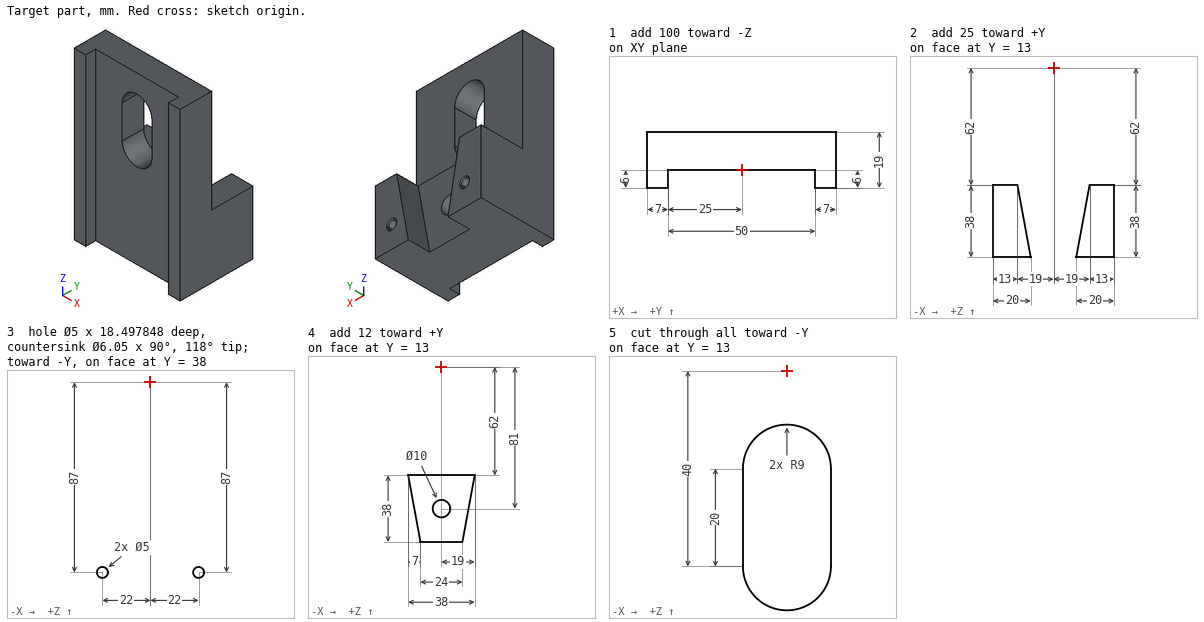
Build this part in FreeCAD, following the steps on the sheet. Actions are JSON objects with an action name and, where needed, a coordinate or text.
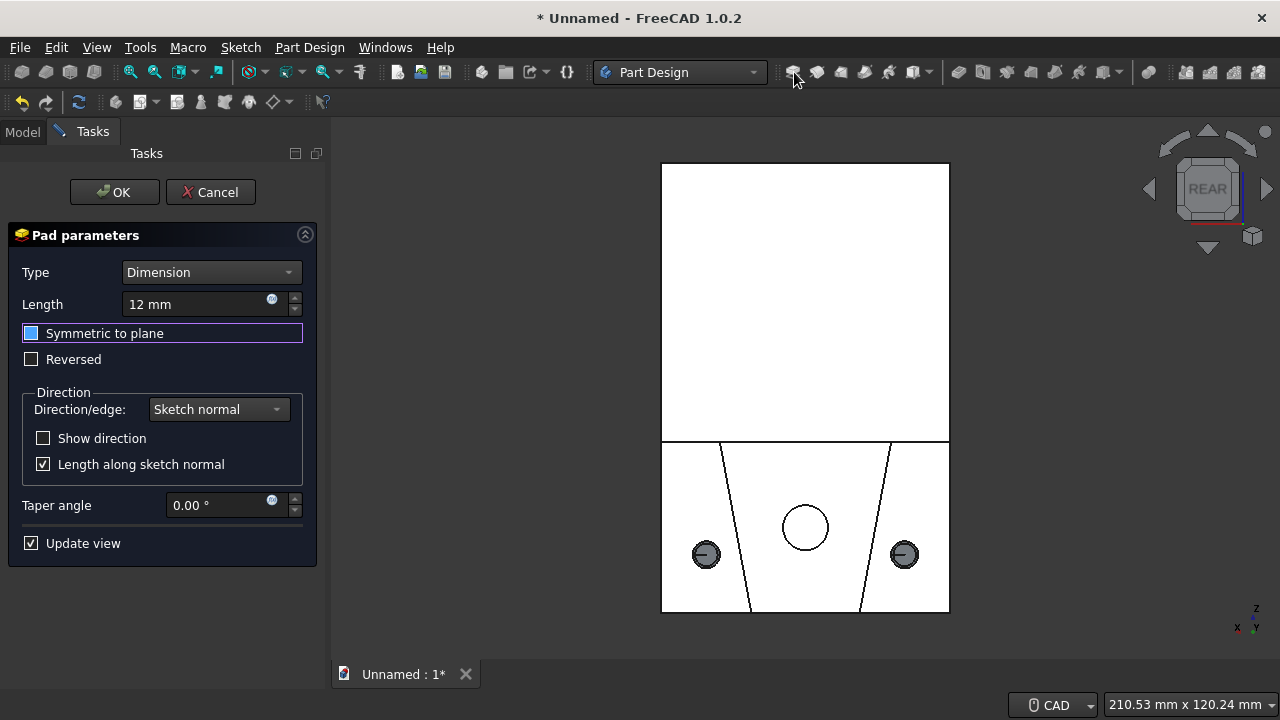
{"action": "left_click", "coordinate": [115, 192]}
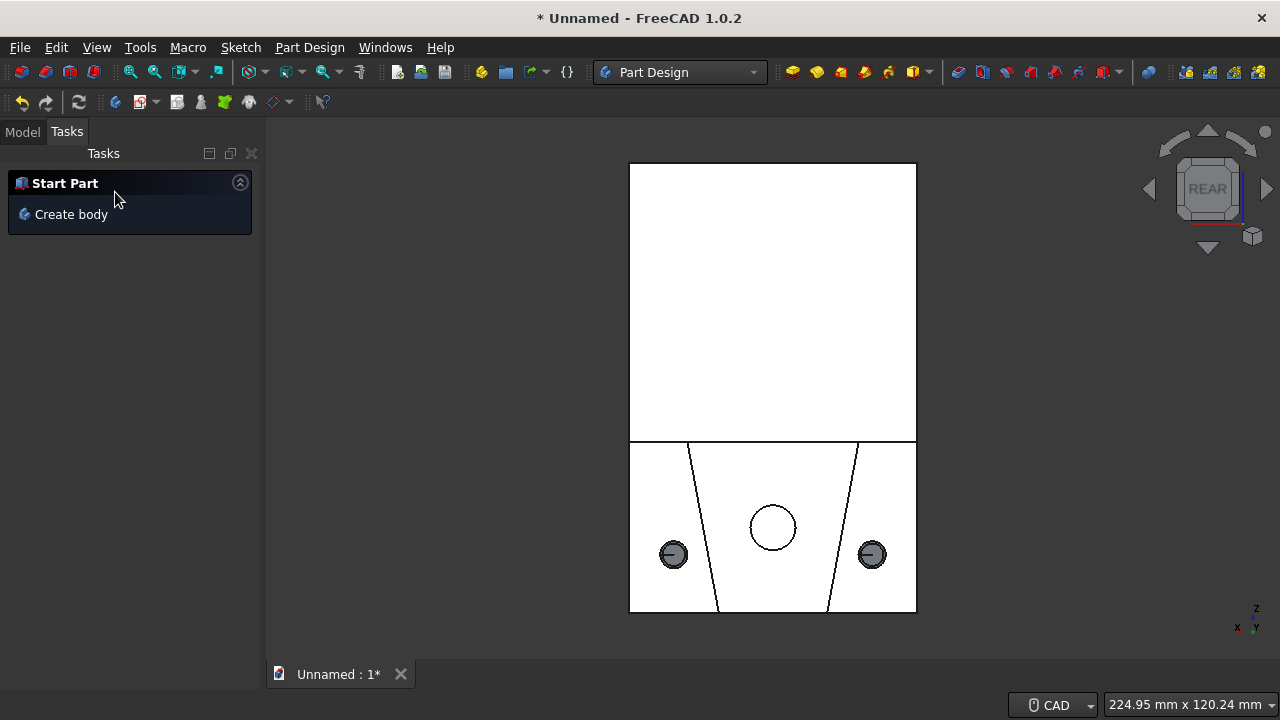
{"action": "left_click", "coordinate": [773, 301]}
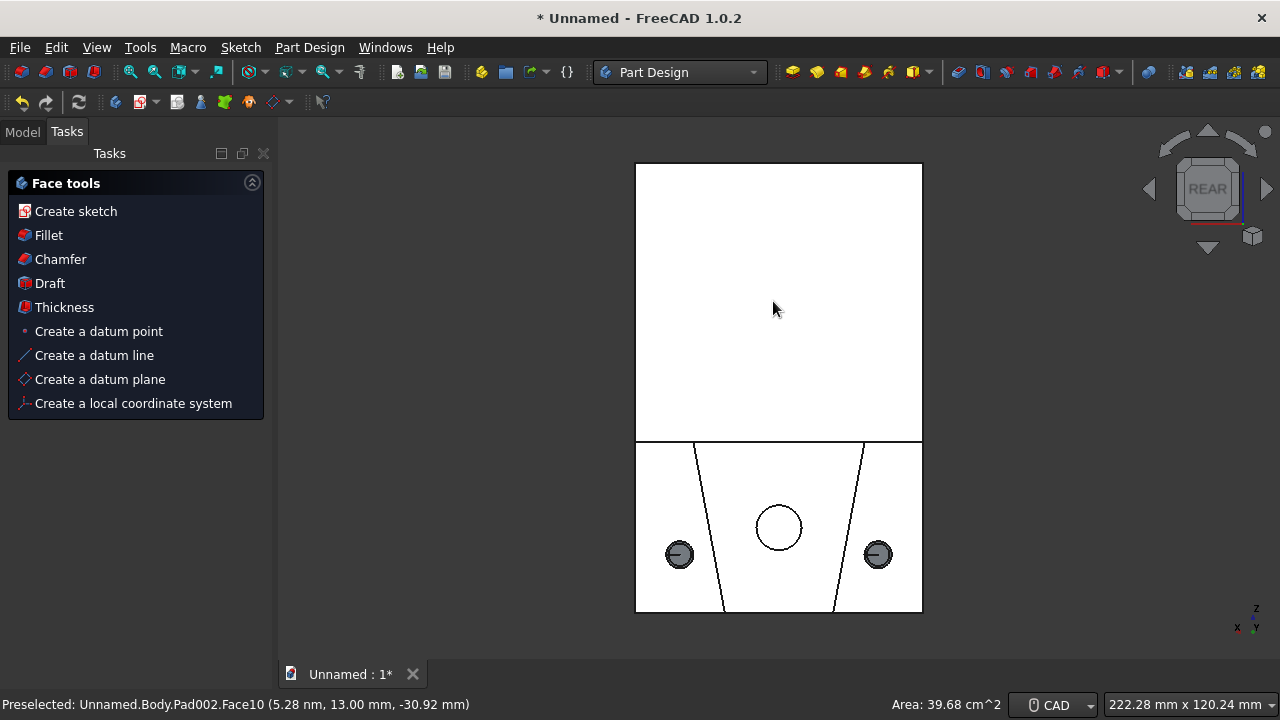
{"action": "left_click", "coordinate": [140, 102]}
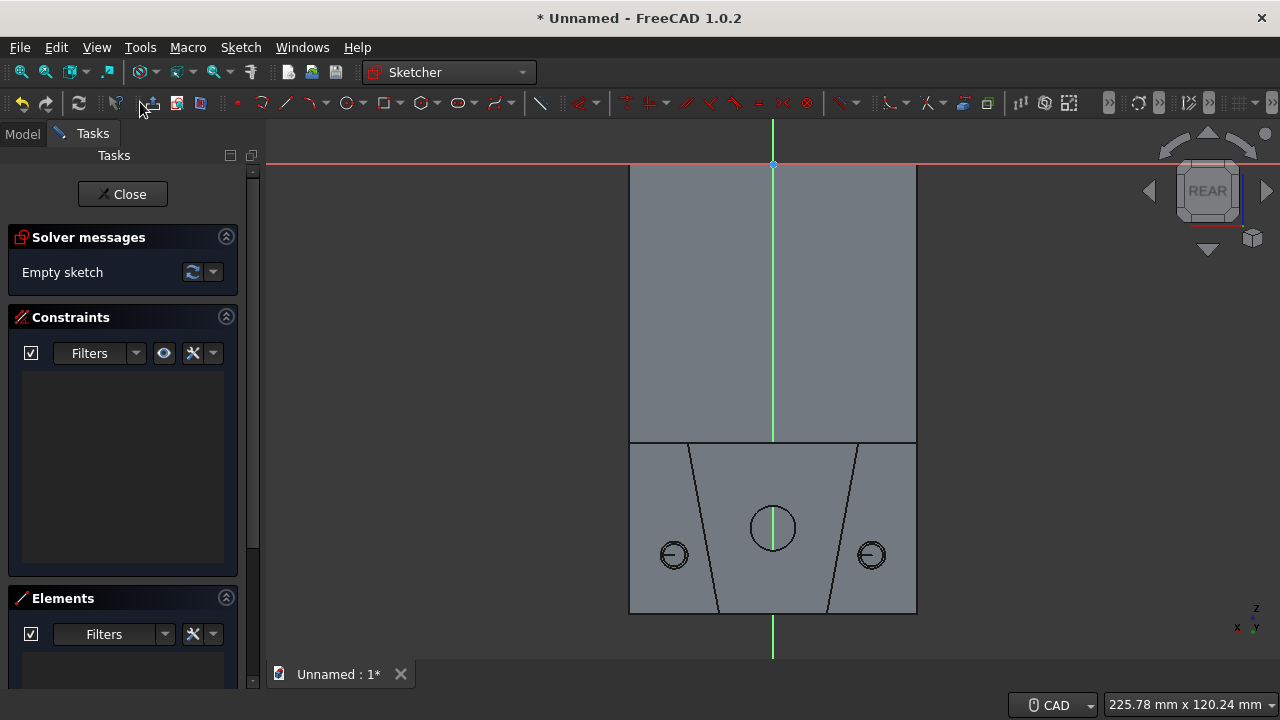
{"action": "key", "text": "q s"}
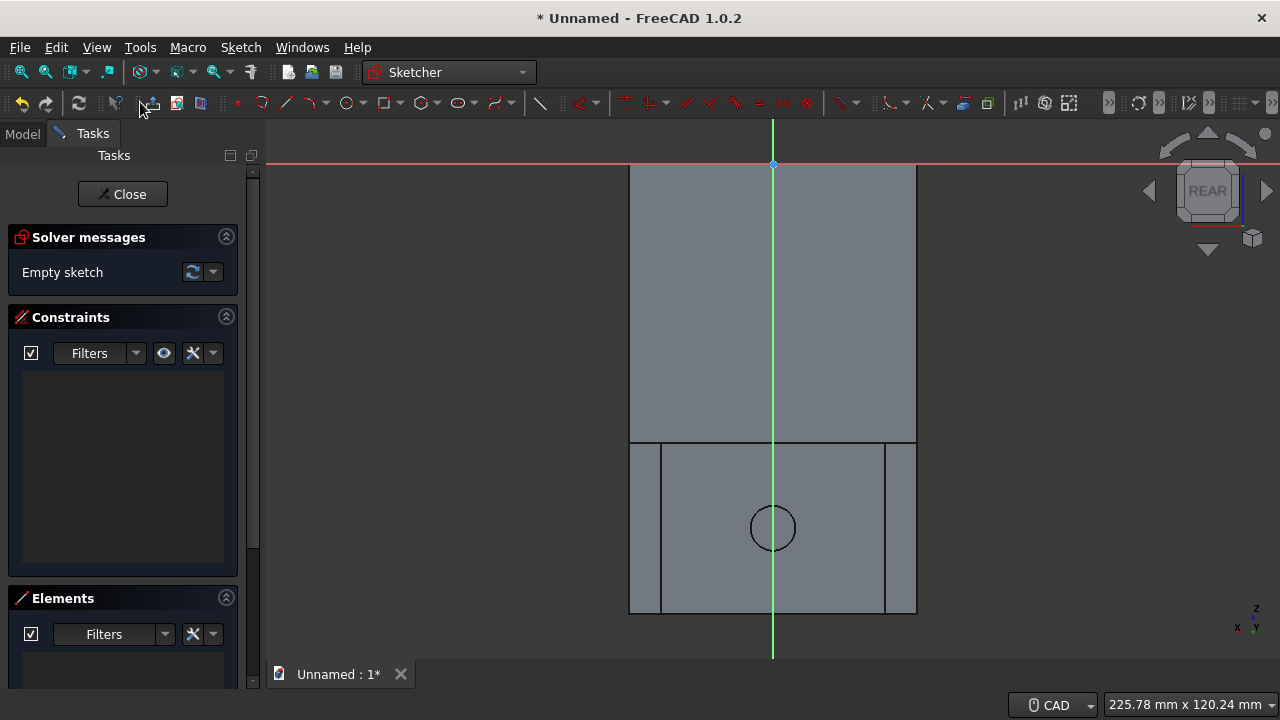
{"action": "scroll", "coordinate": [912, 147], "scroll_direction": "up", "scroll_amount": 2}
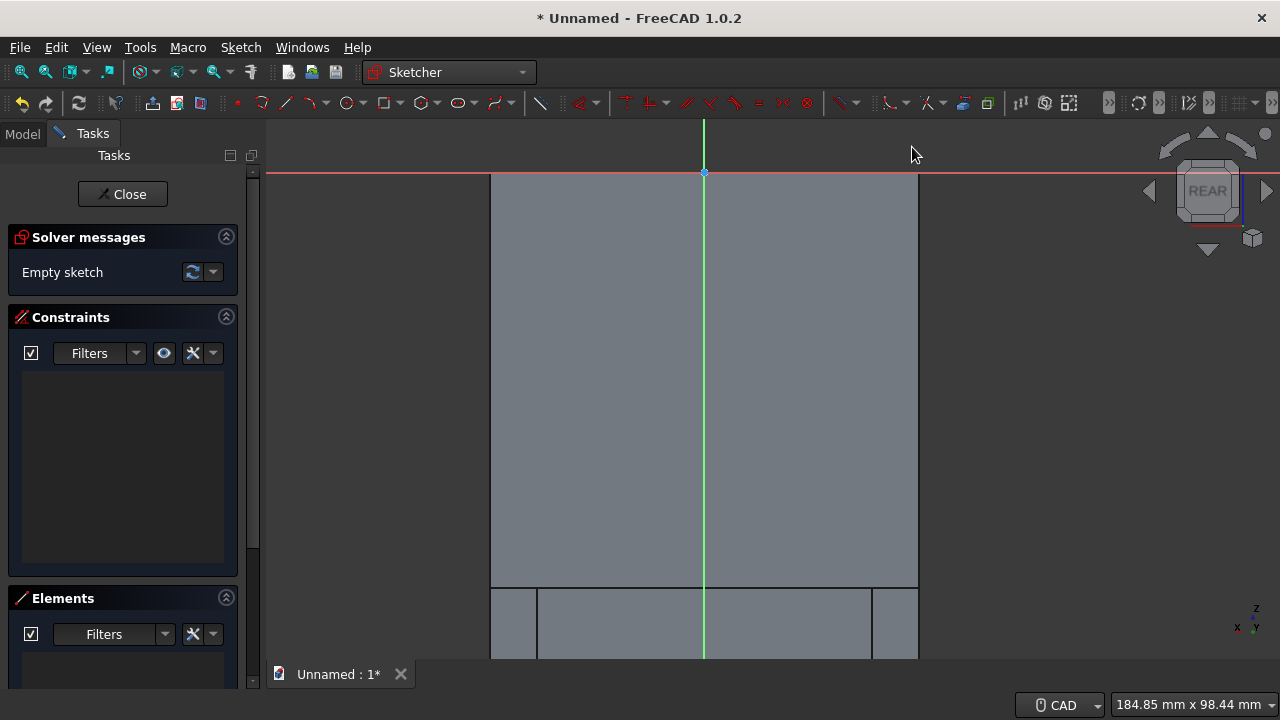
{"action": "left_click", "coordinate": [458, 104]}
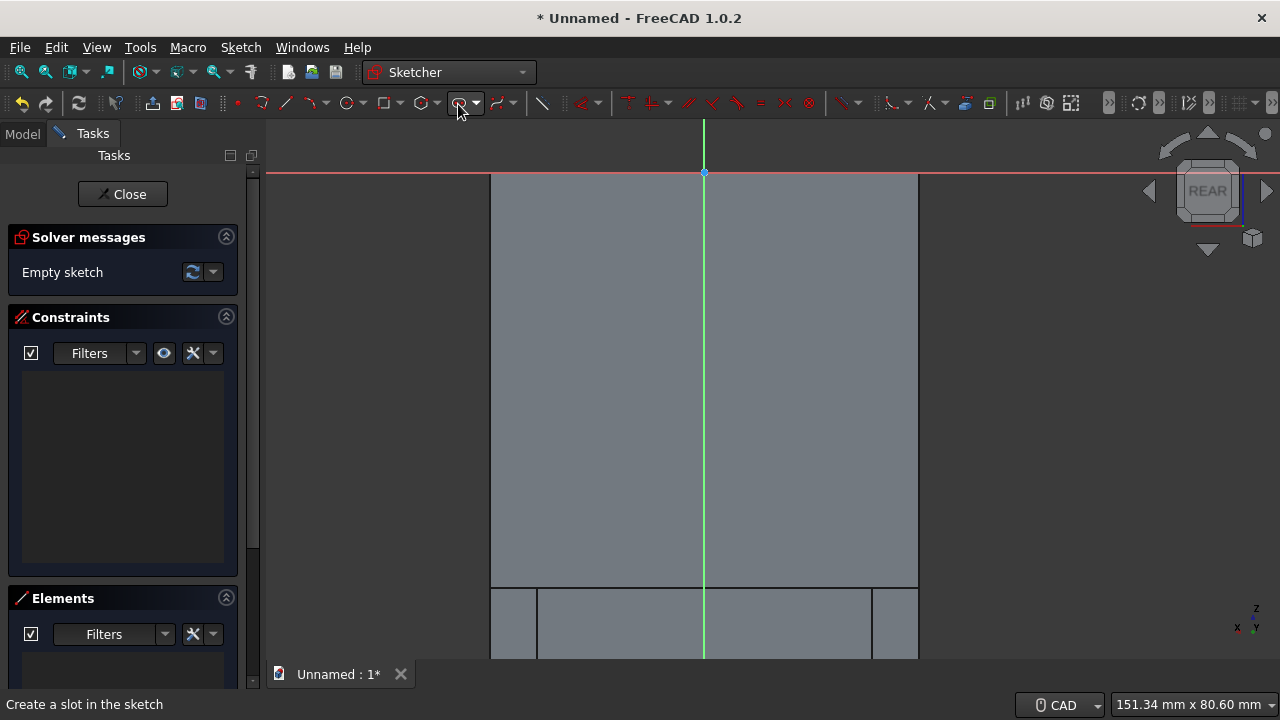
{"action": "left_click", "coordinate": [704, 441]}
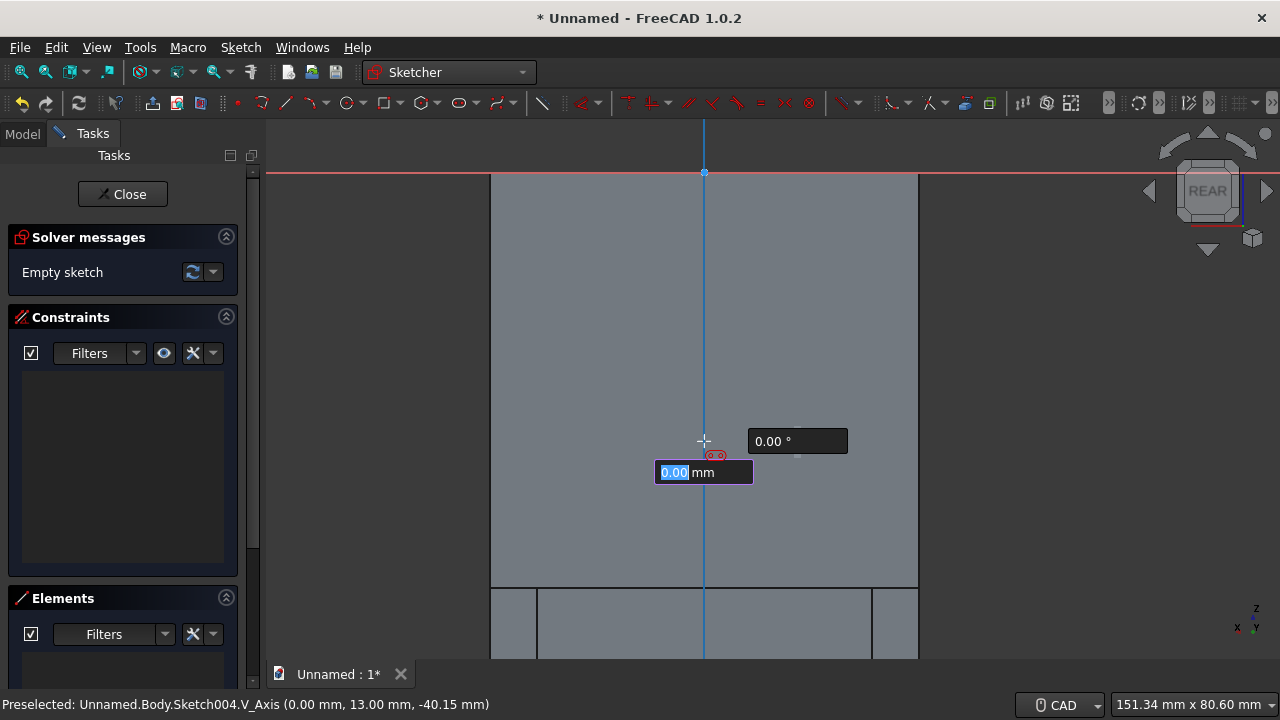
{"action": "left_click", "coordinate": [713, 307]}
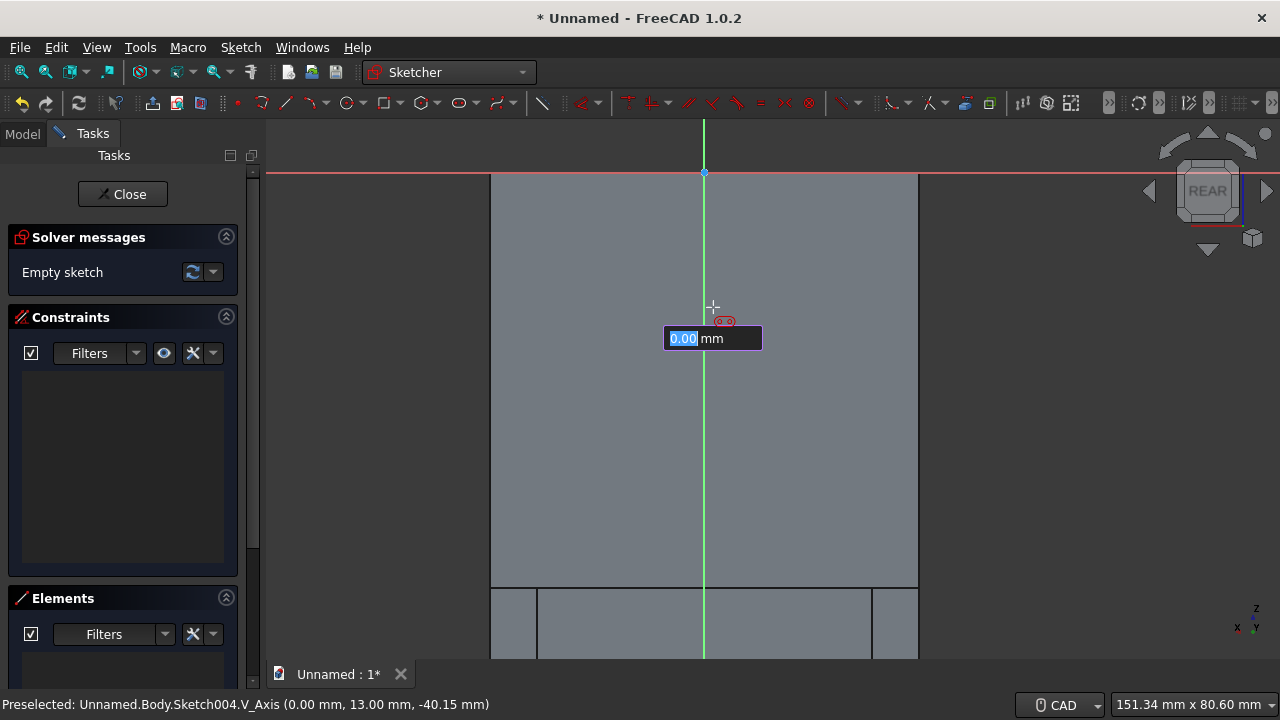
{"action": "left_click", "coordinate": [765, 374]}
{"action": "key", "text": "Escape"}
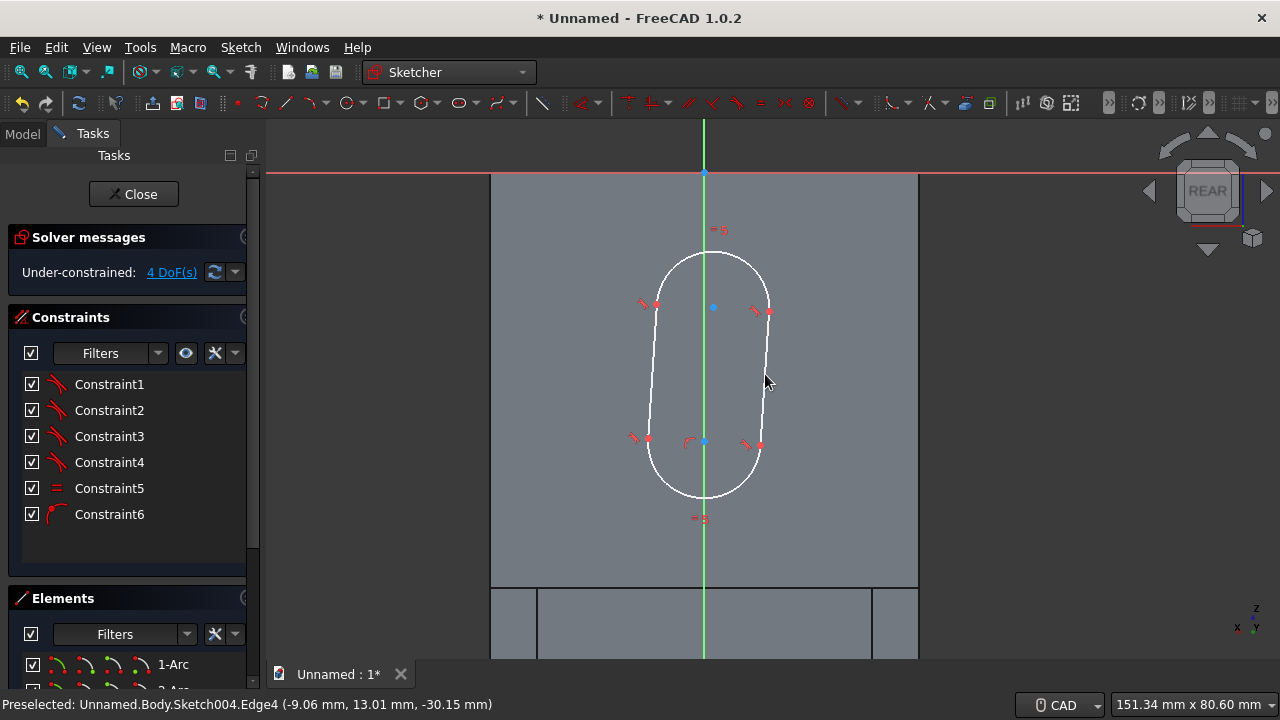
{"action": "left_click", "coordinate": [651, 398]}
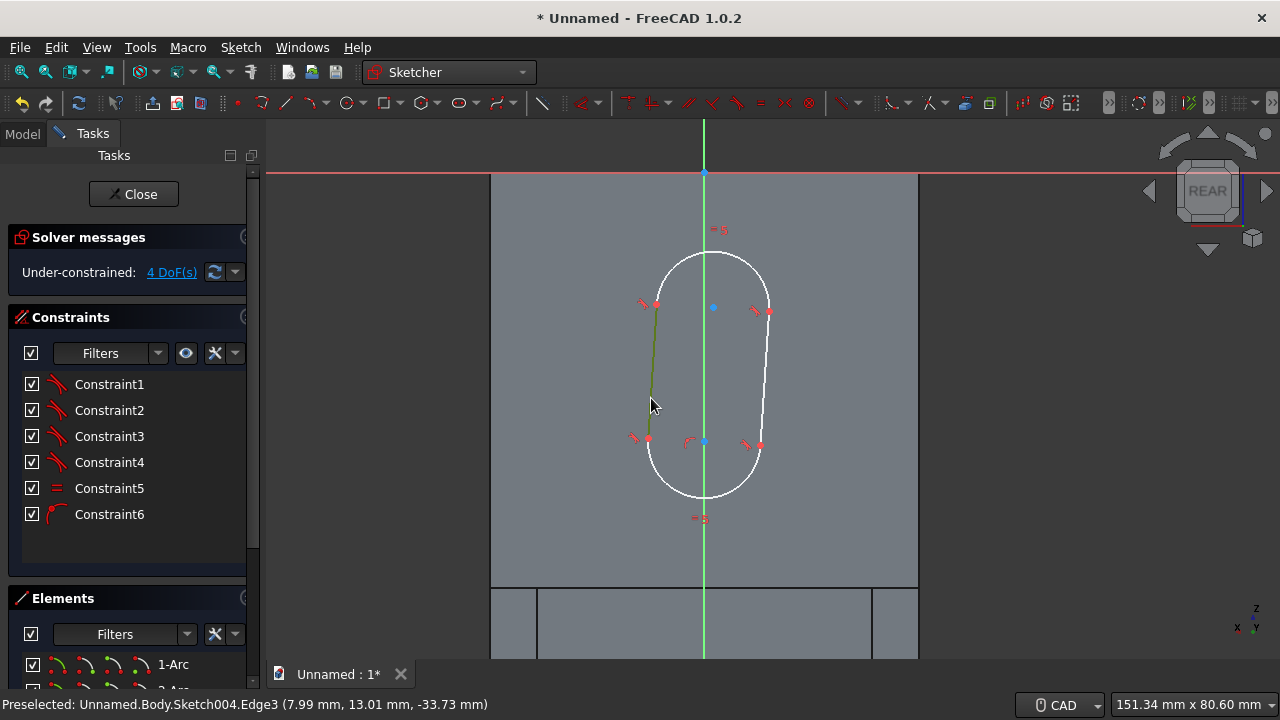
{"action": "key", "text": "v"}